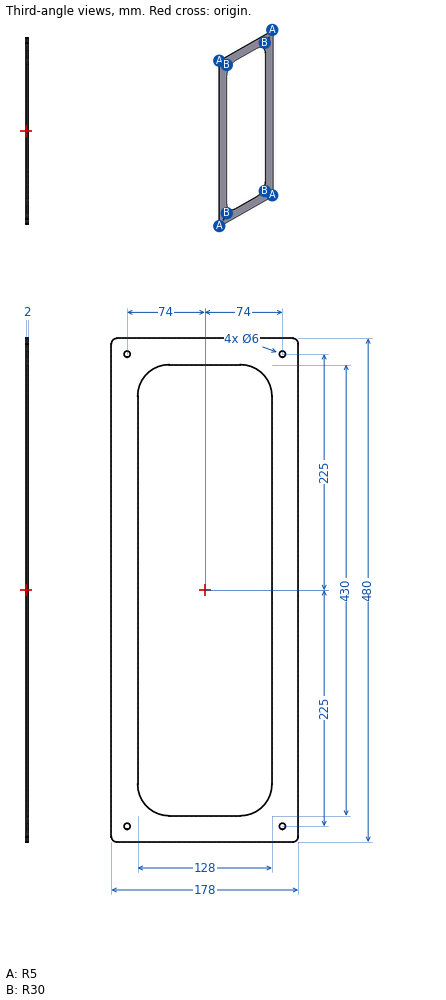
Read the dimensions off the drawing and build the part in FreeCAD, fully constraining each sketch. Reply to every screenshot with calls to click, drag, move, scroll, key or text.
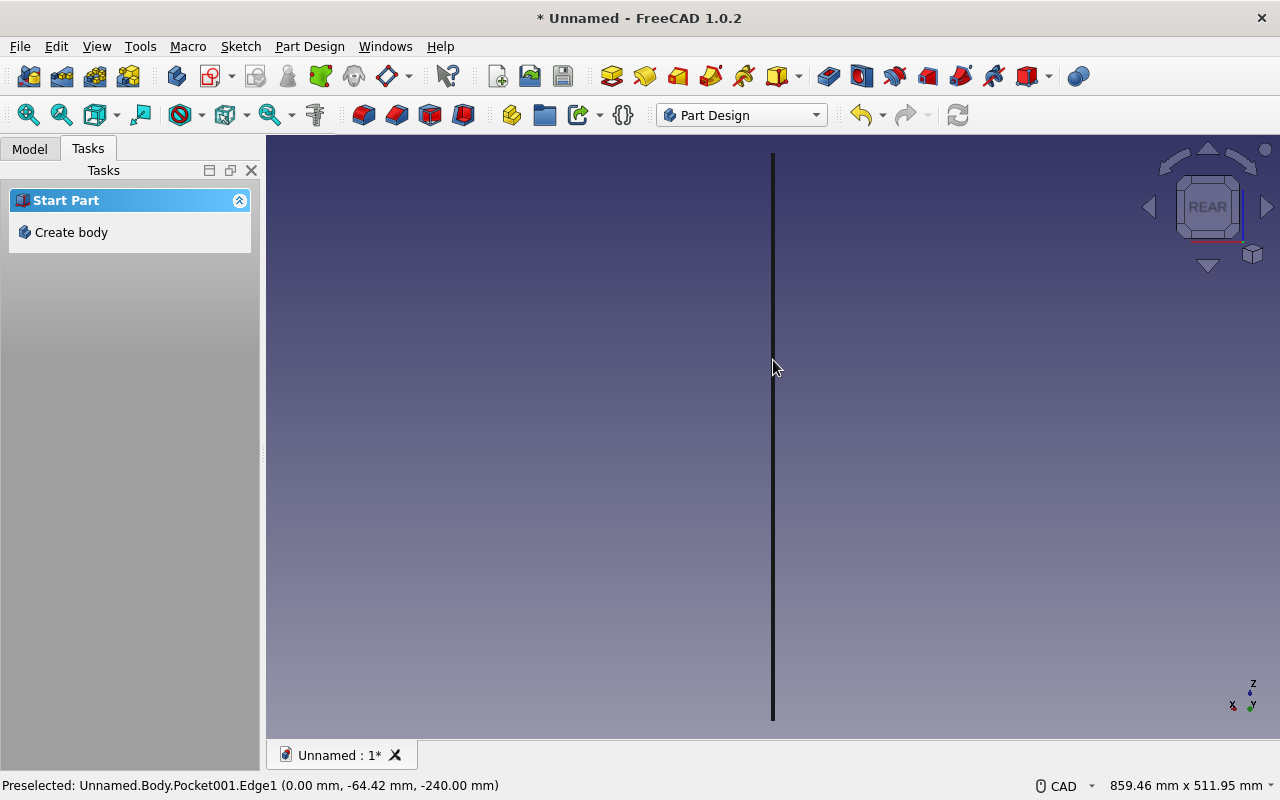
scroll(773, 182, up, 15)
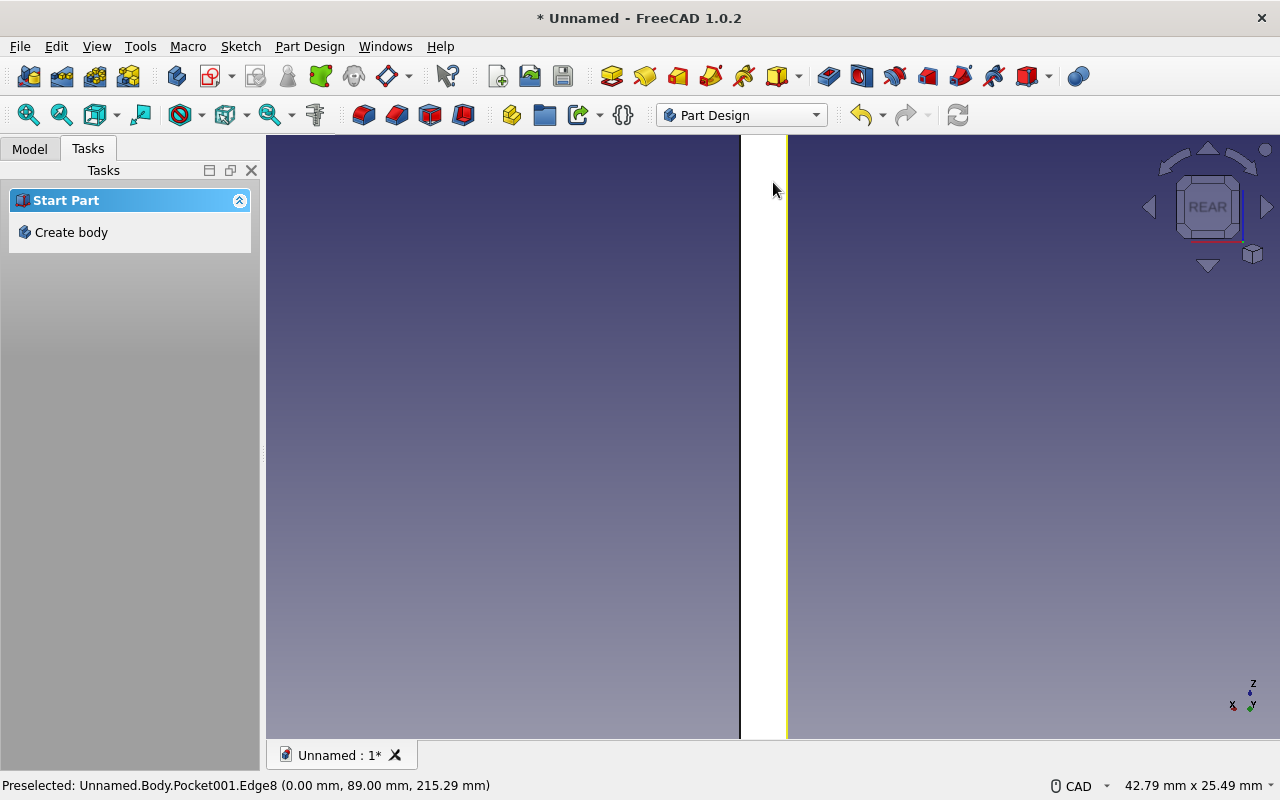
key(v)
key(f)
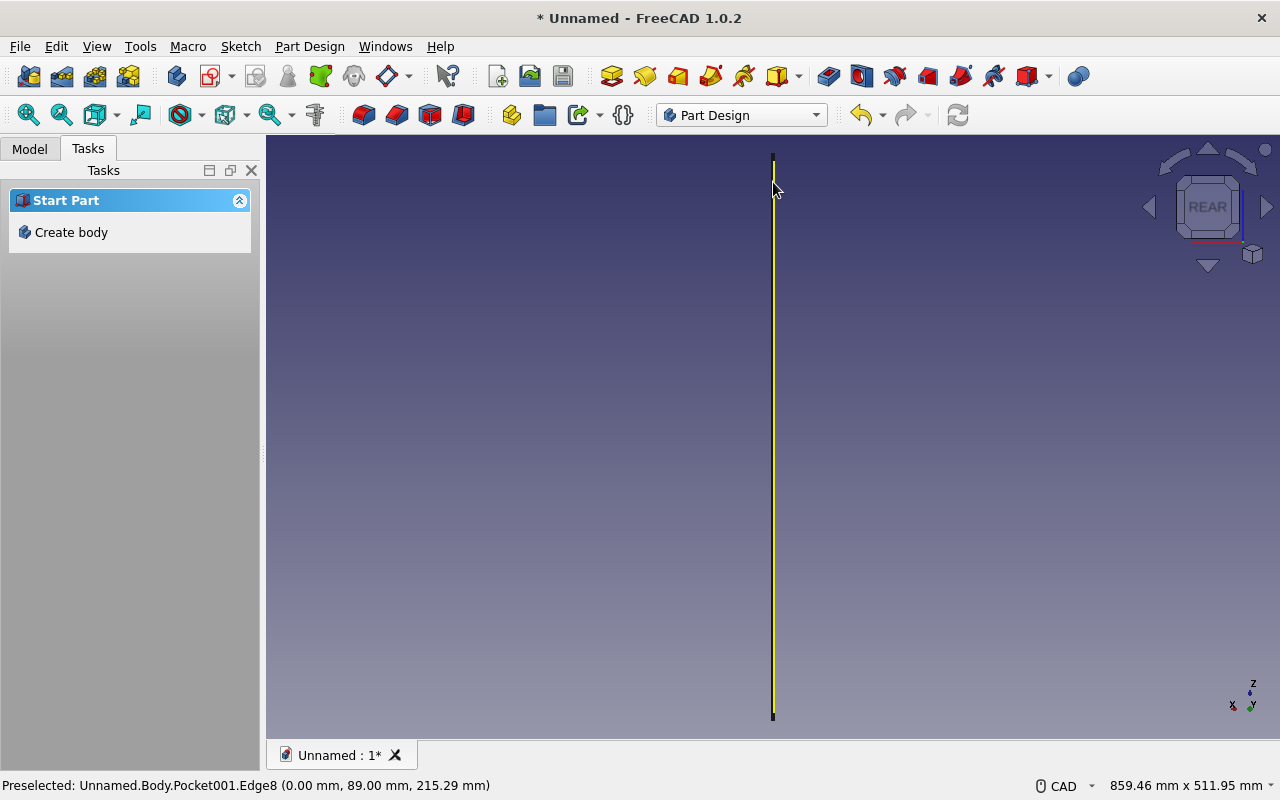
key(6)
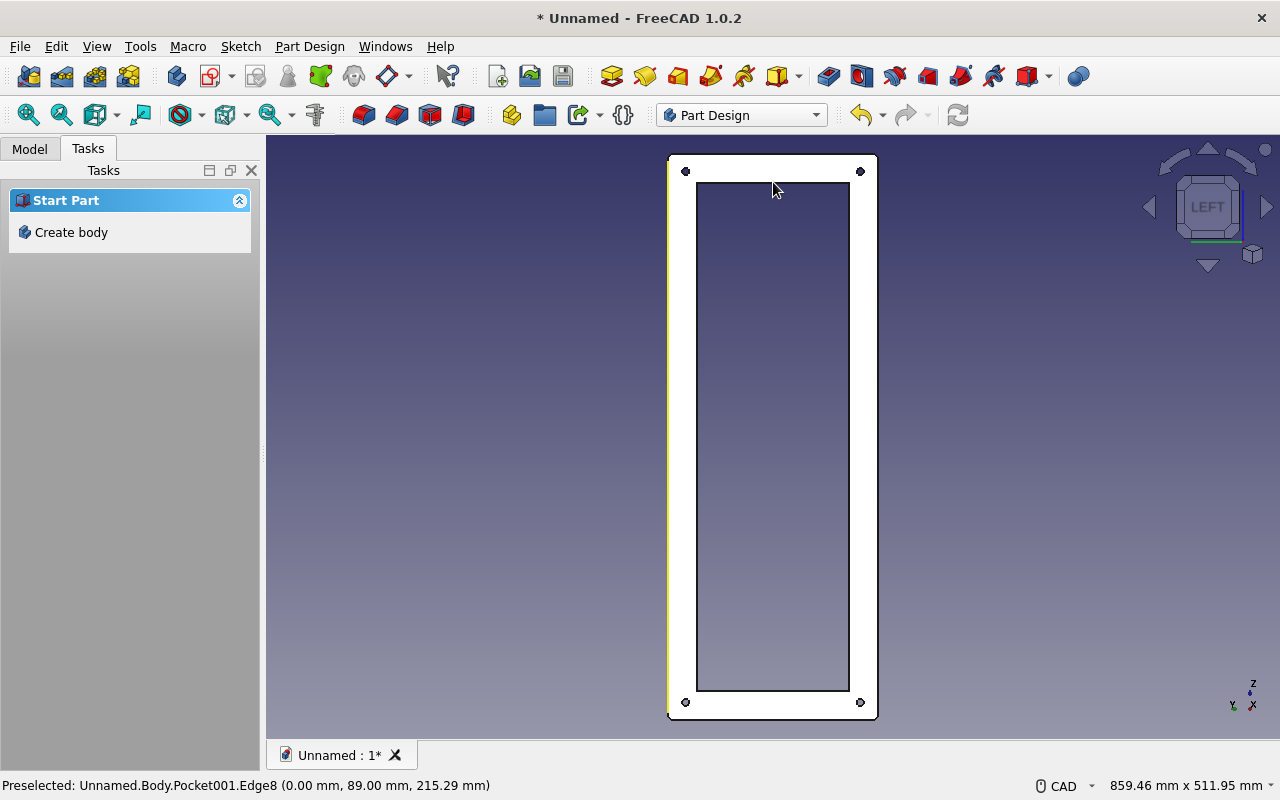
scroll(849, 182, up, 15)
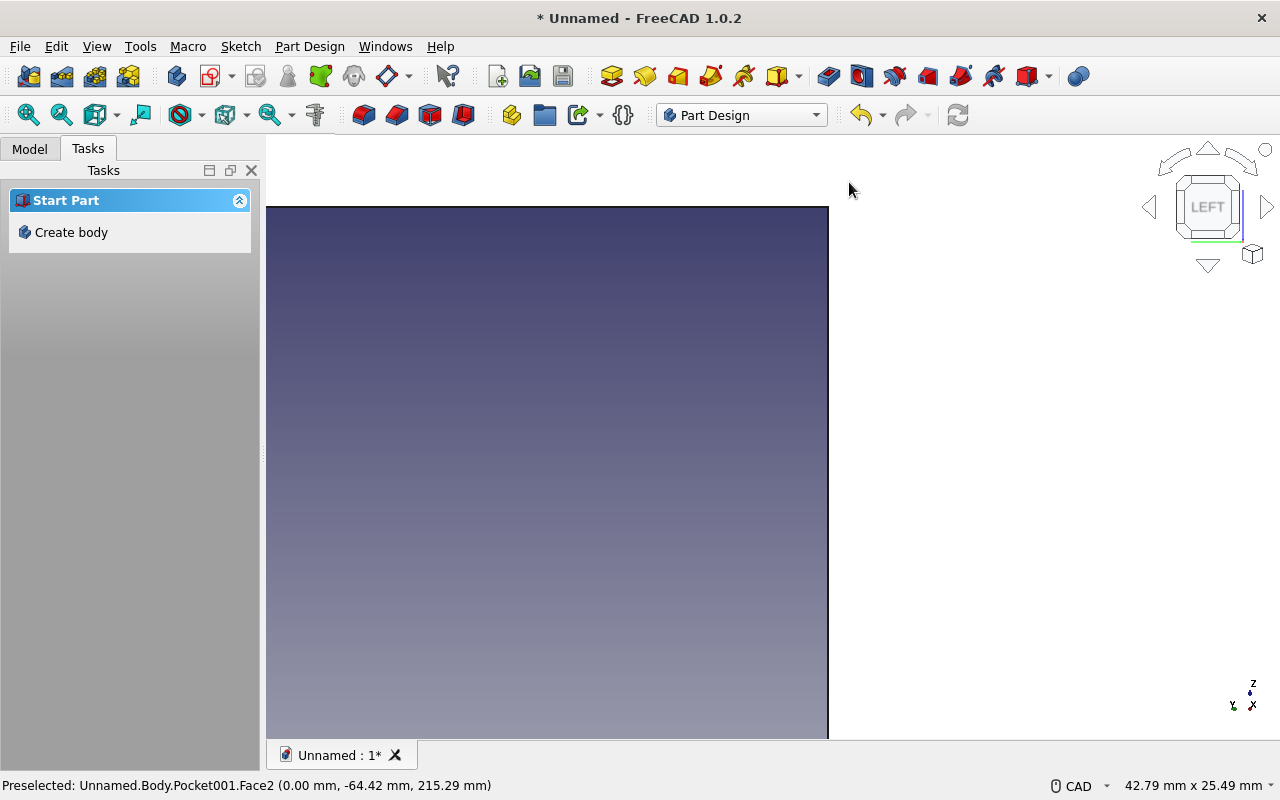
key(v)
key(f)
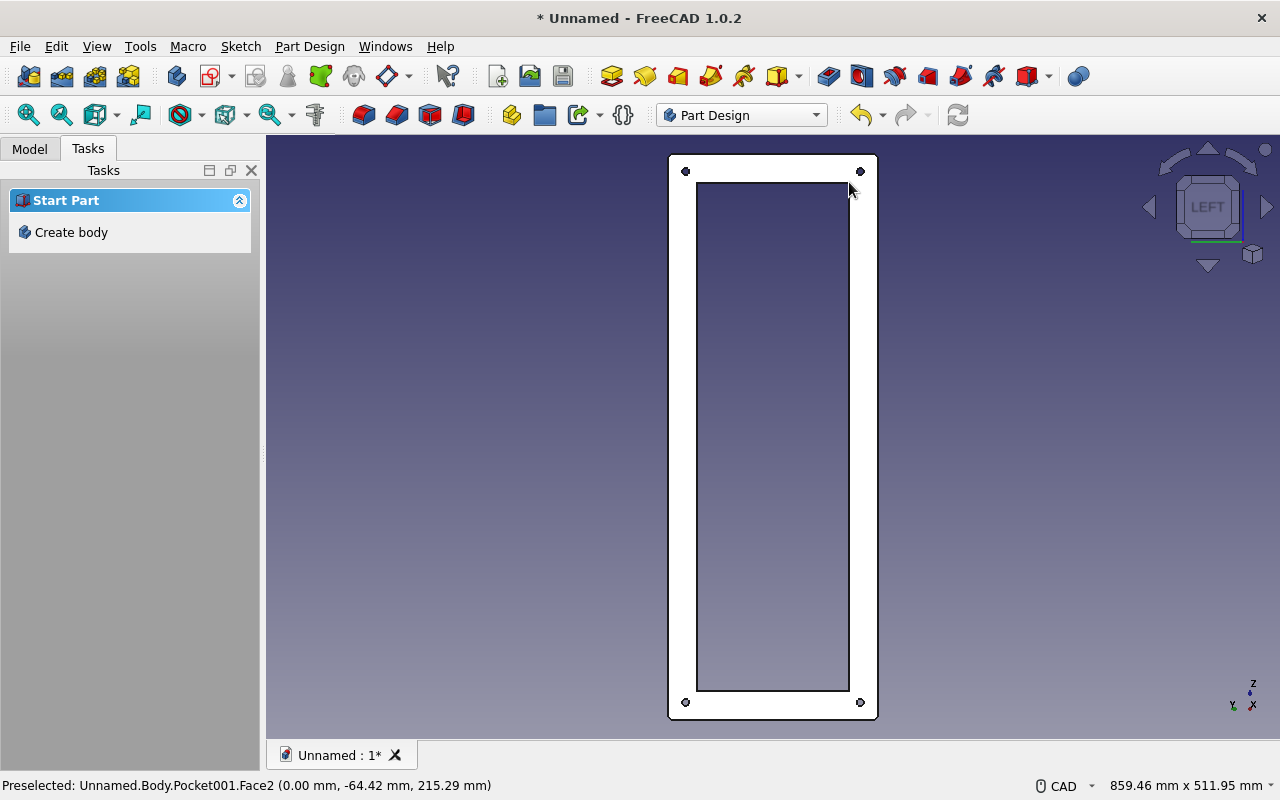
key(v)
key(3)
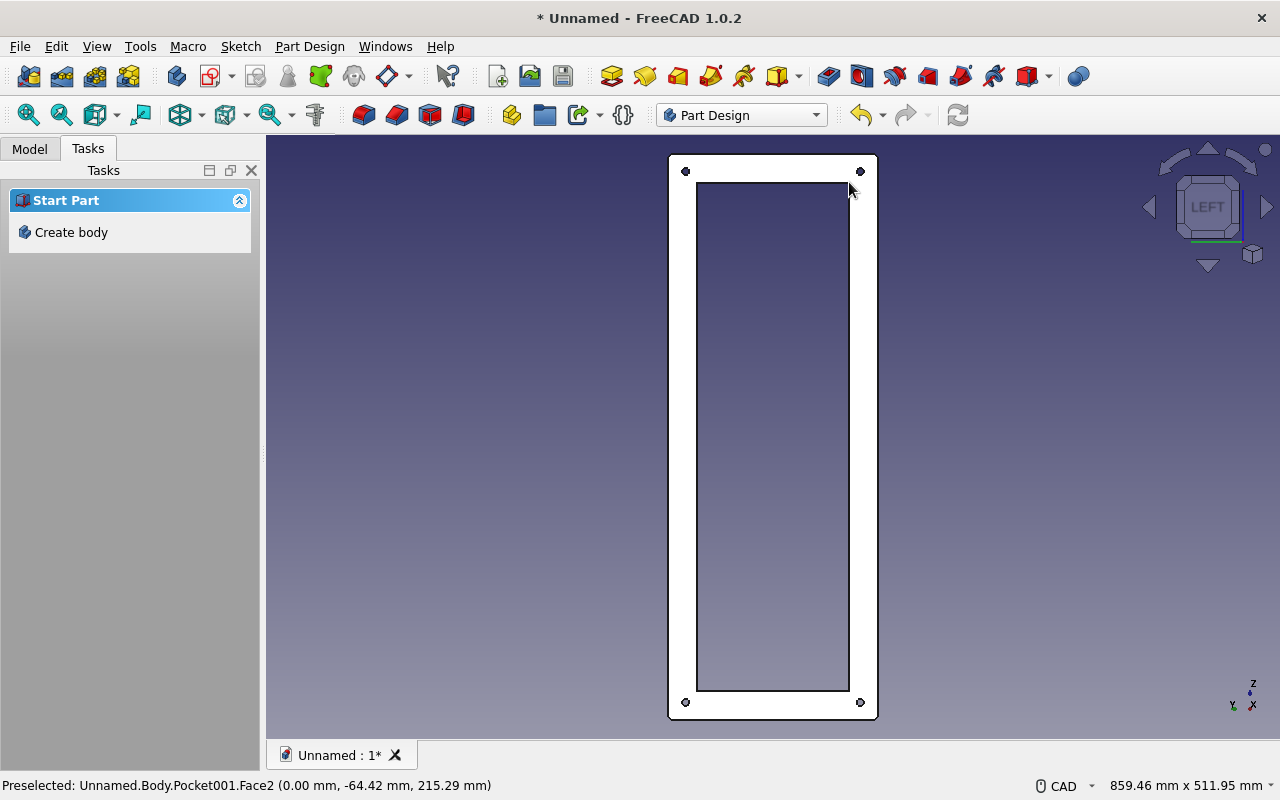
key(0)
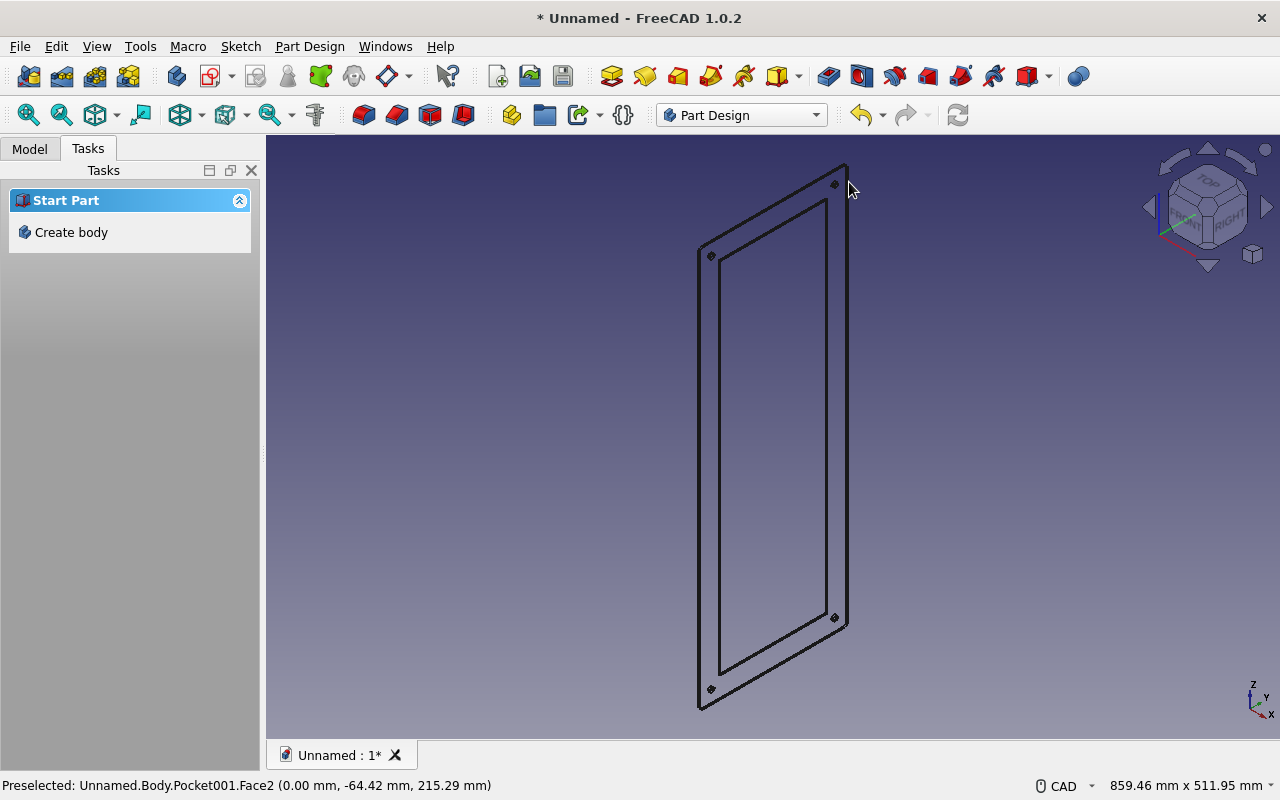
scroll(720, 260, up, 15)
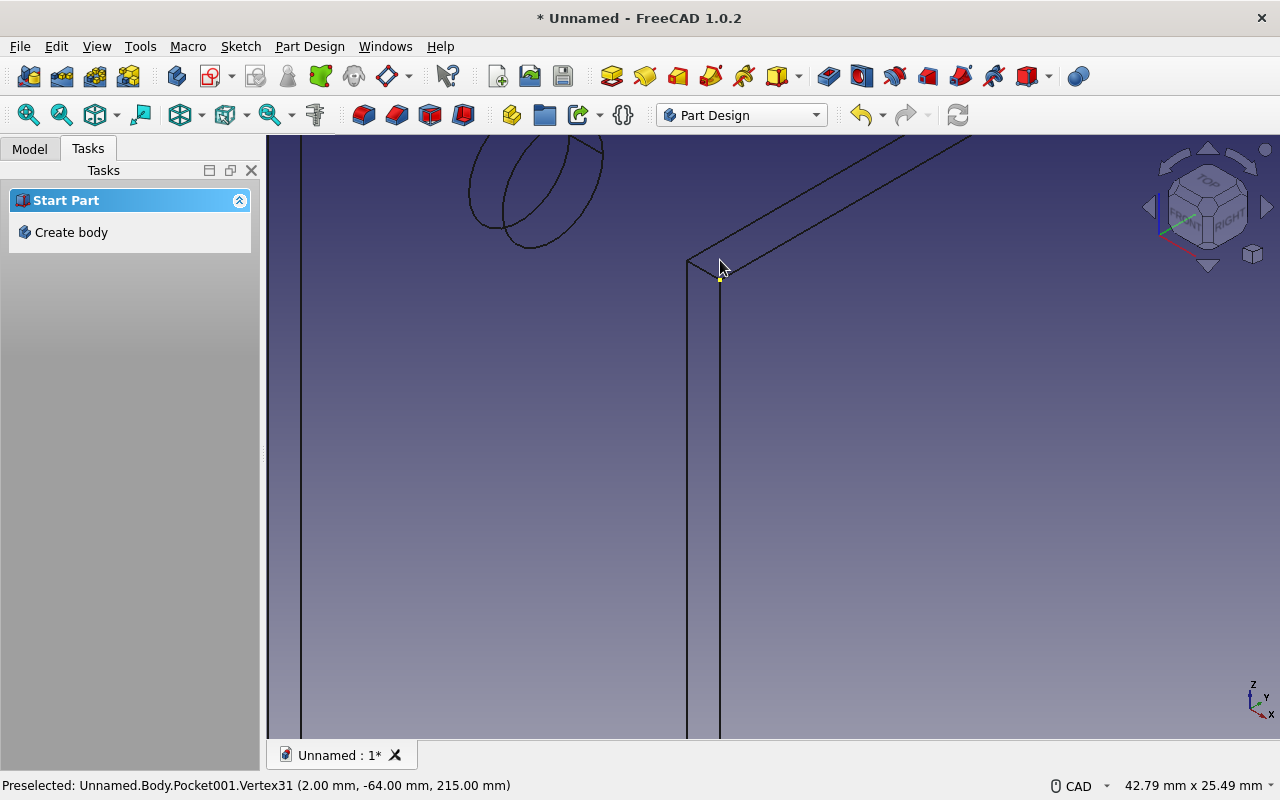
click(704, 269)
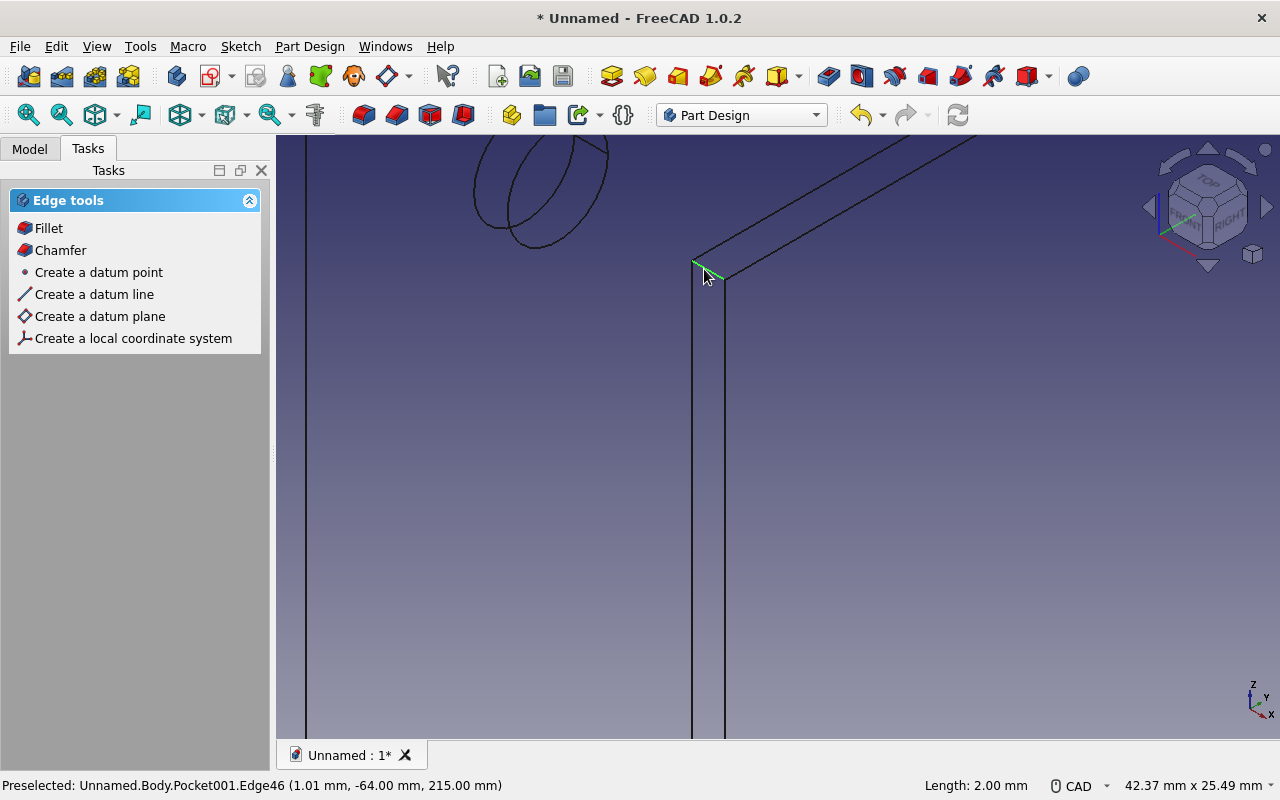
key(v)
key(f)